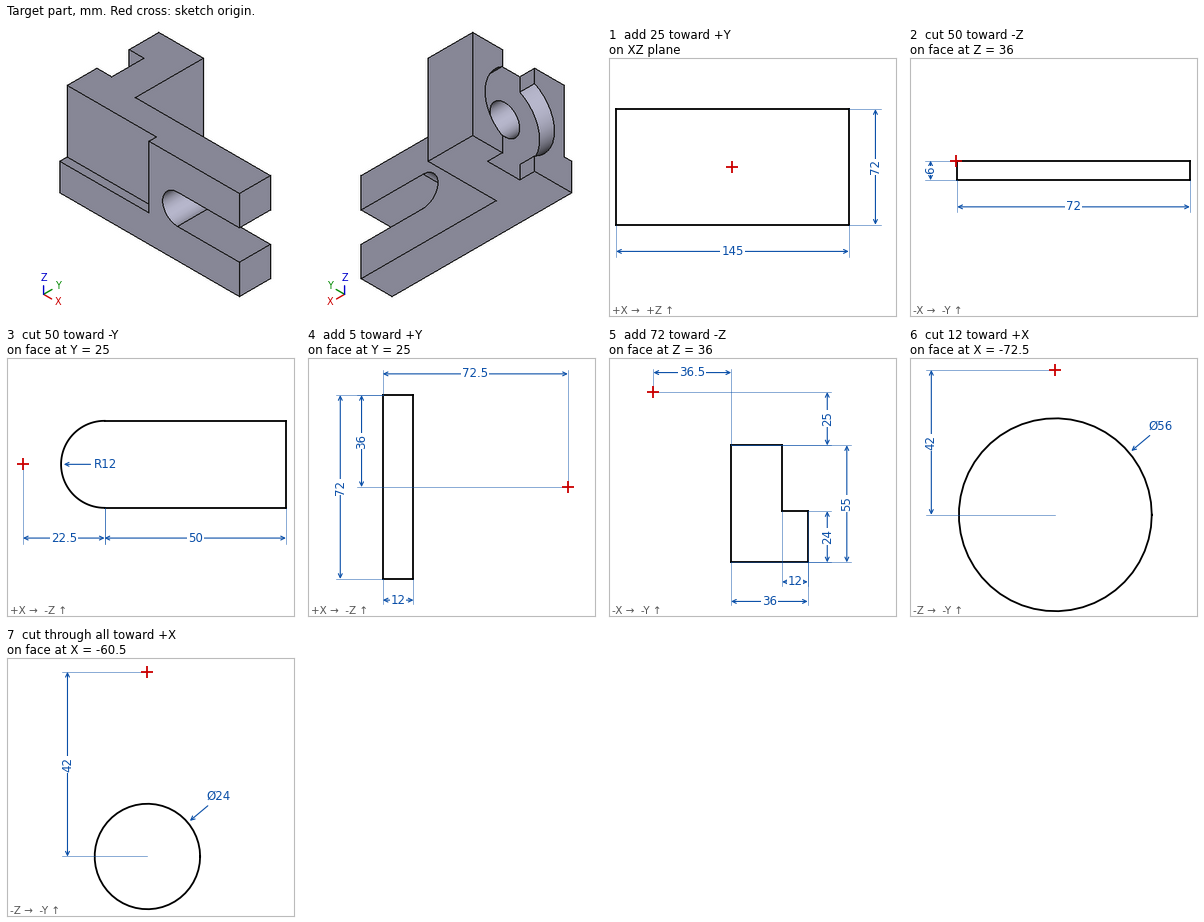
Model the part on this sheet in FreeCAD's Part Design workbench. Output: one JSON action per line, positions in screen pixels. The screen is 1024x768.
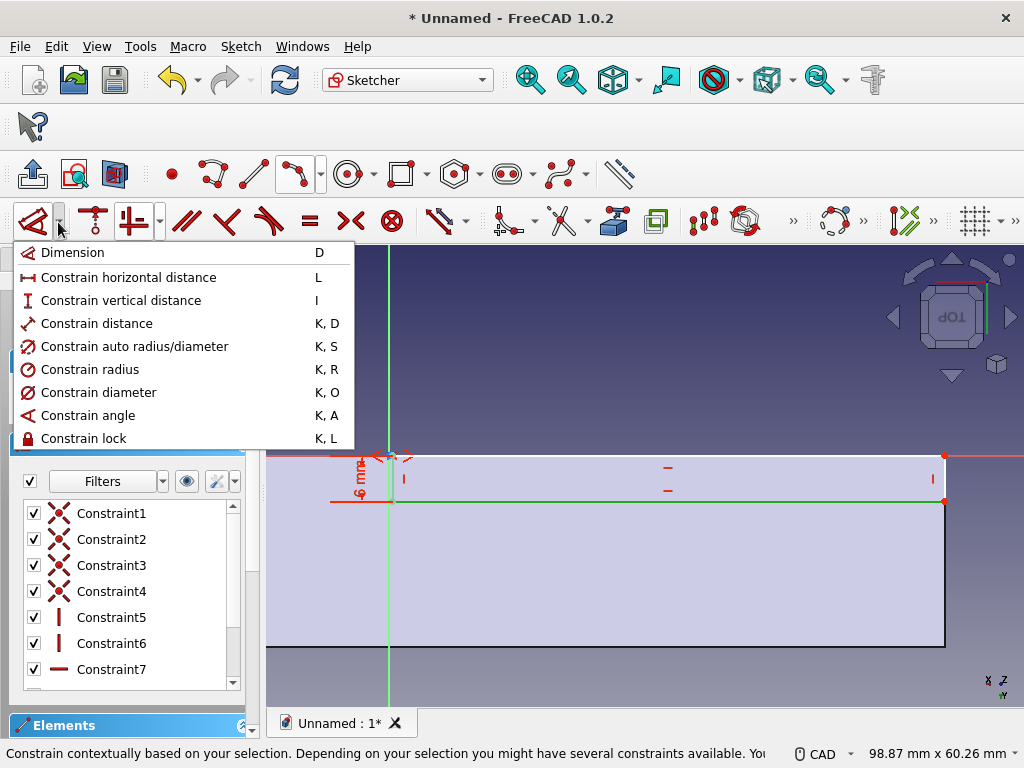
{"action": "left_click", "coordinate": [184, 278]}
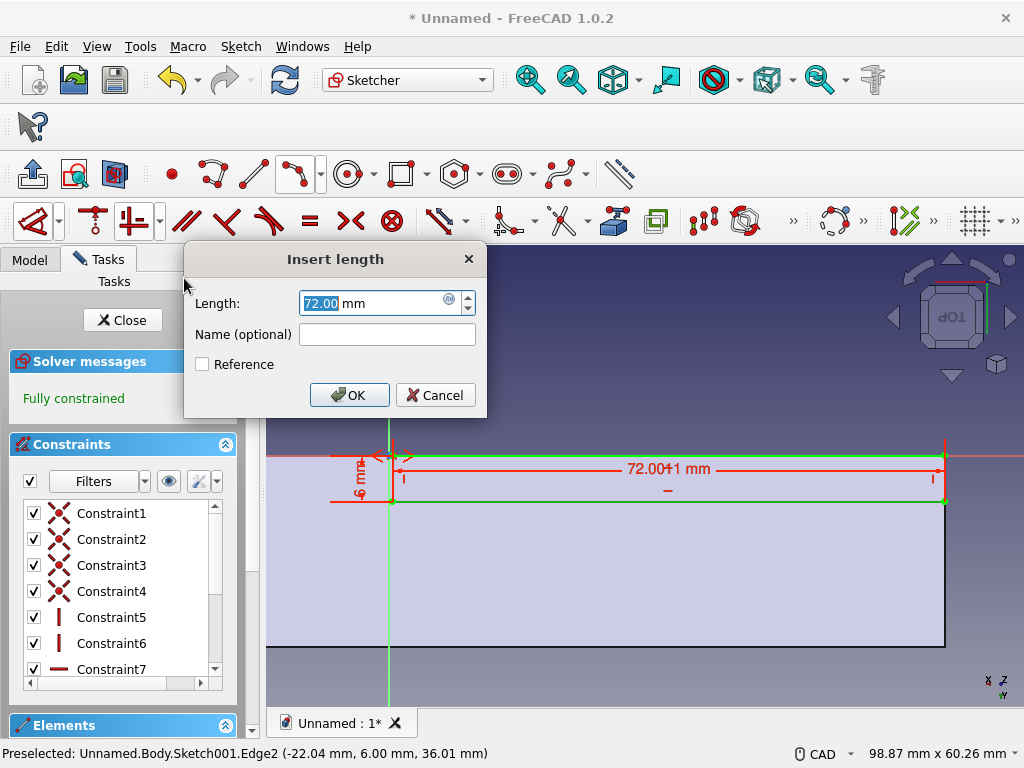
{"action": "type", "text": "72"}
{"action": "key", "text": "Return"}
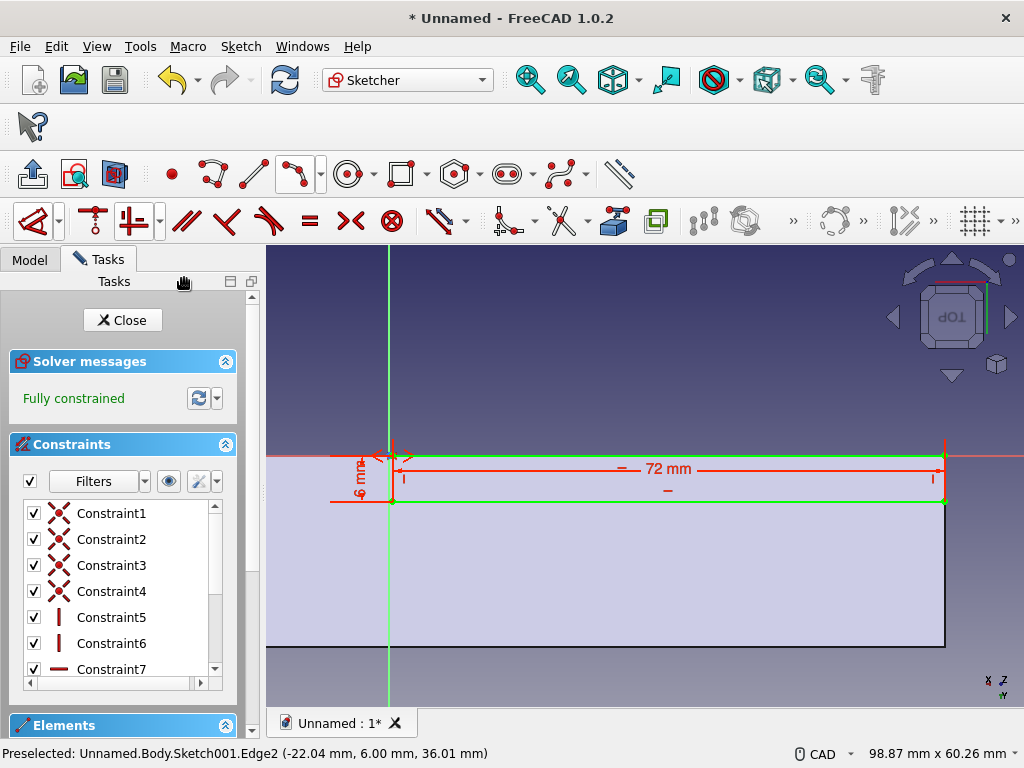
{"action": "left_click", "coordinate": [123, 320]}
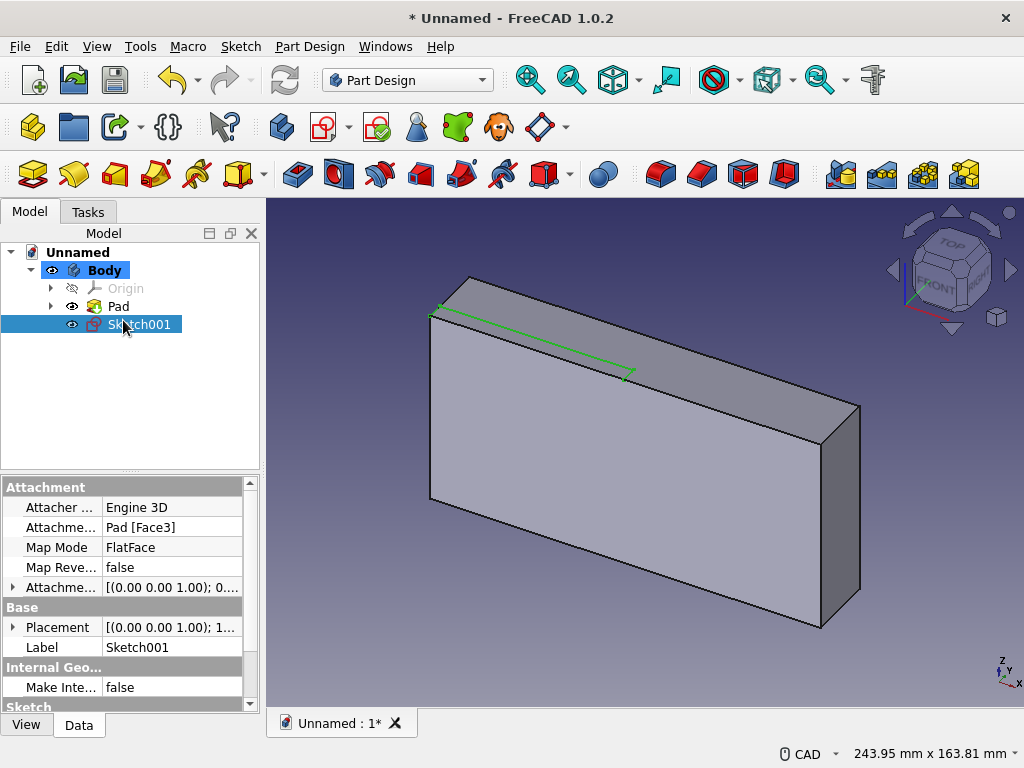
{"action": "left_click", "coordinate": [298, 174]}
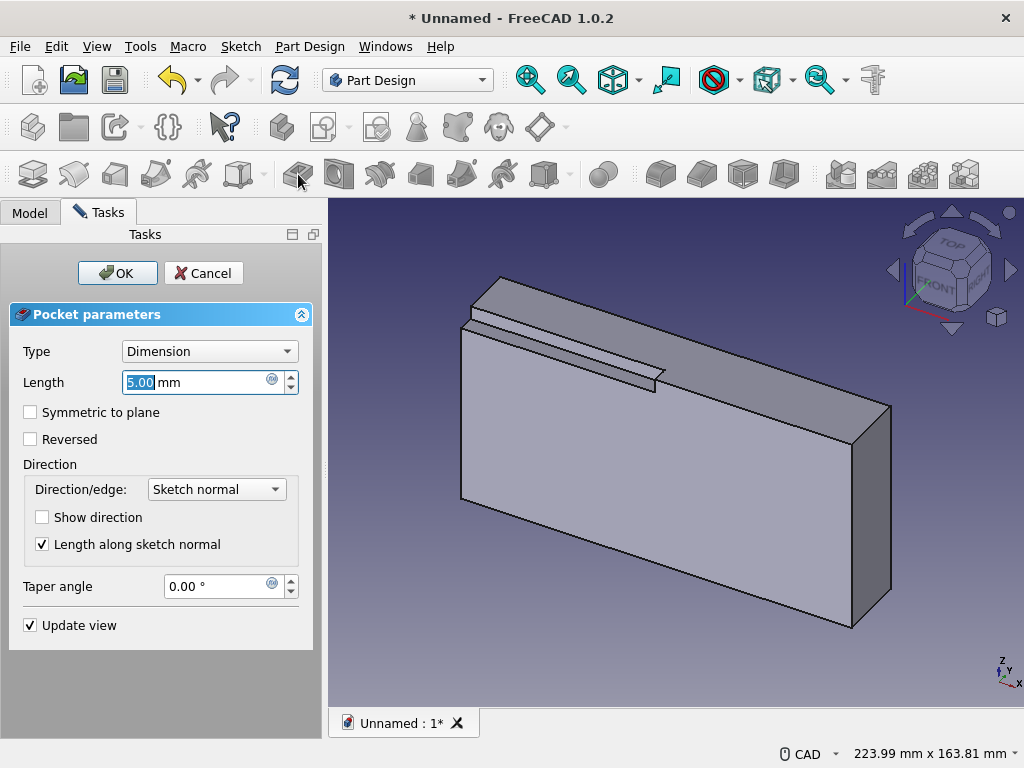
{"action": "type", "text": "50"}
{"action": "key", "text": "Tab"}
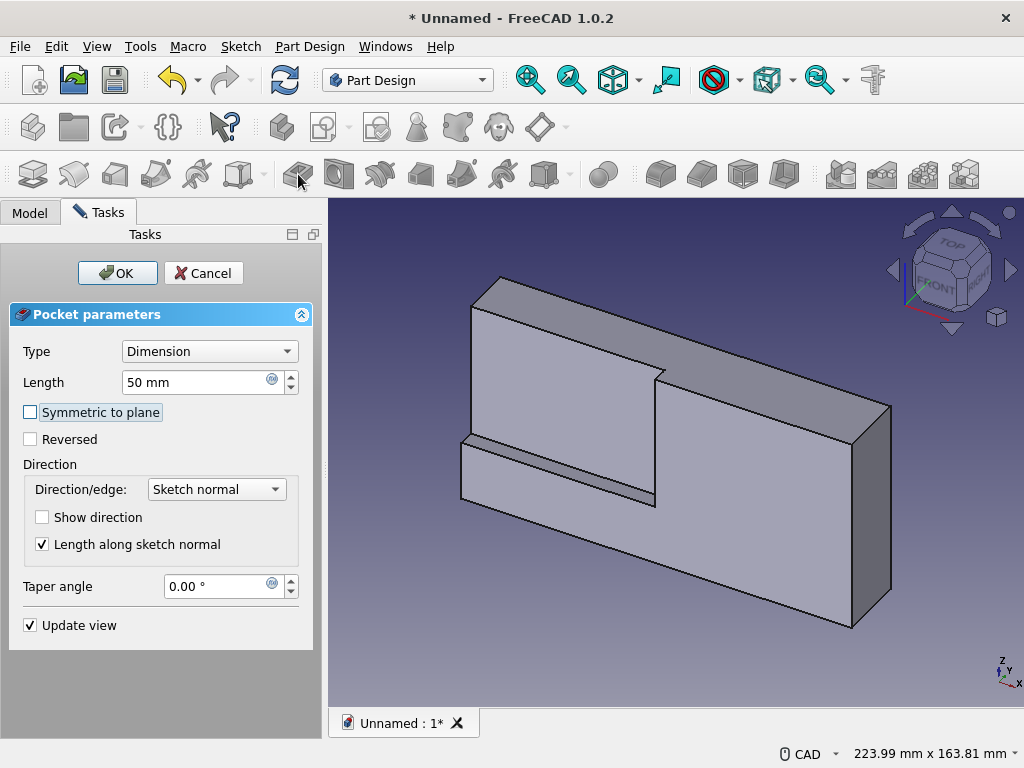
{"action": "left_click", "coordinate": [118, 273]}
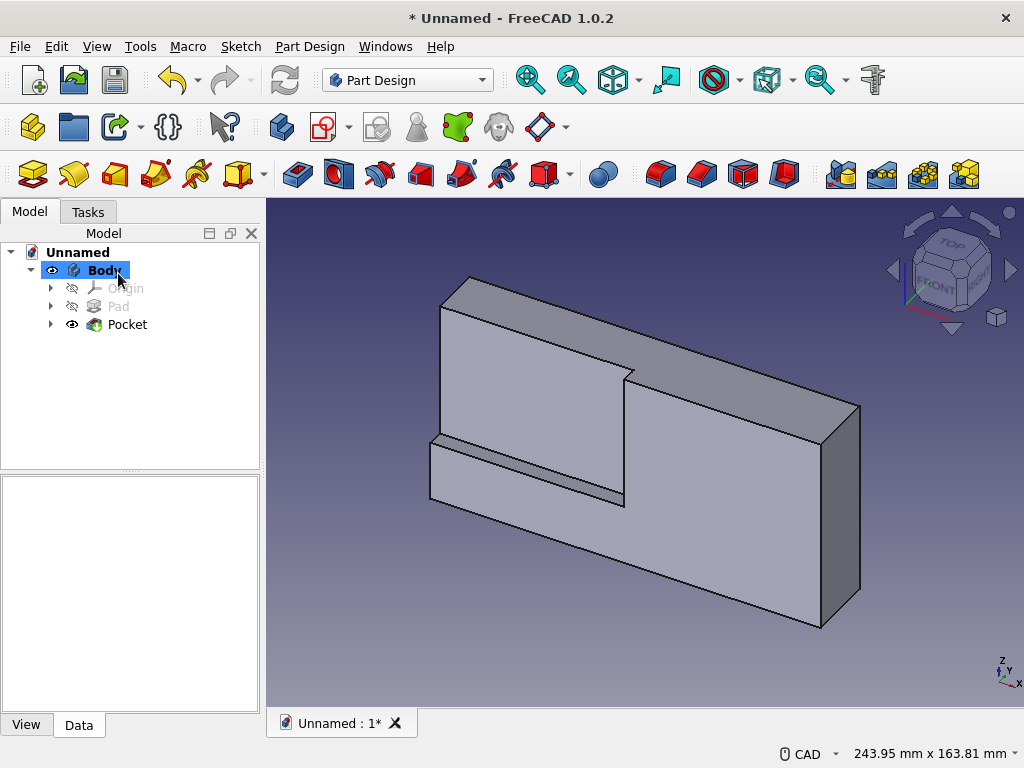
{"action": "key", "text": "4"}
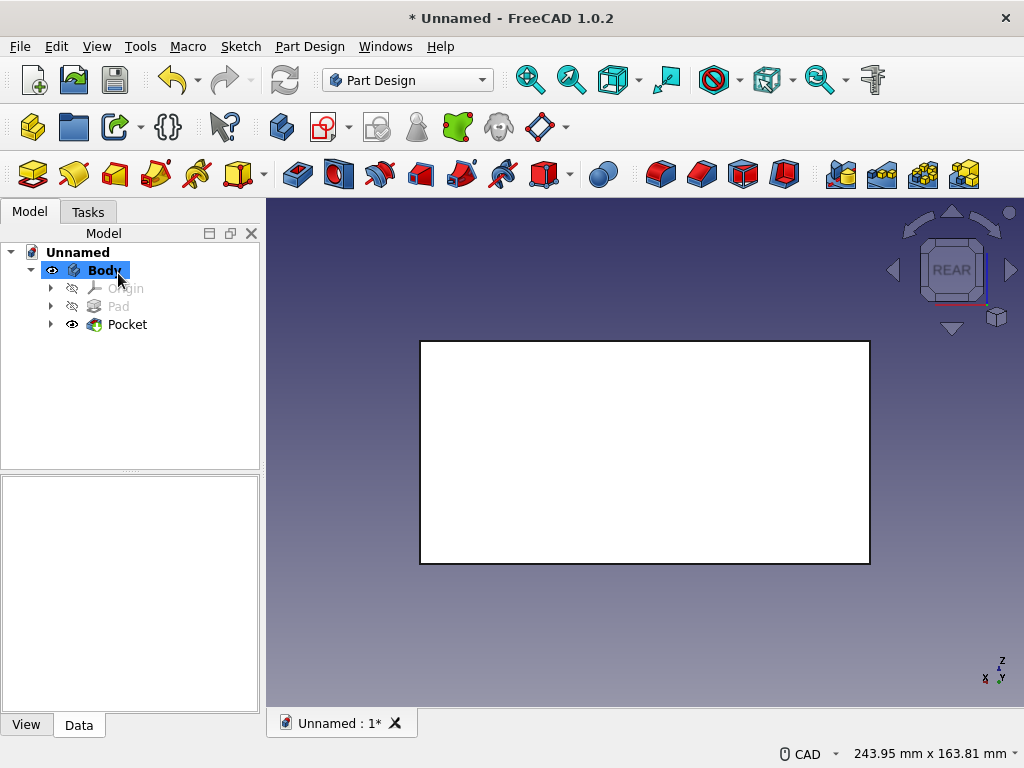
{"action": "left_click", "coordinate": [581, 452]}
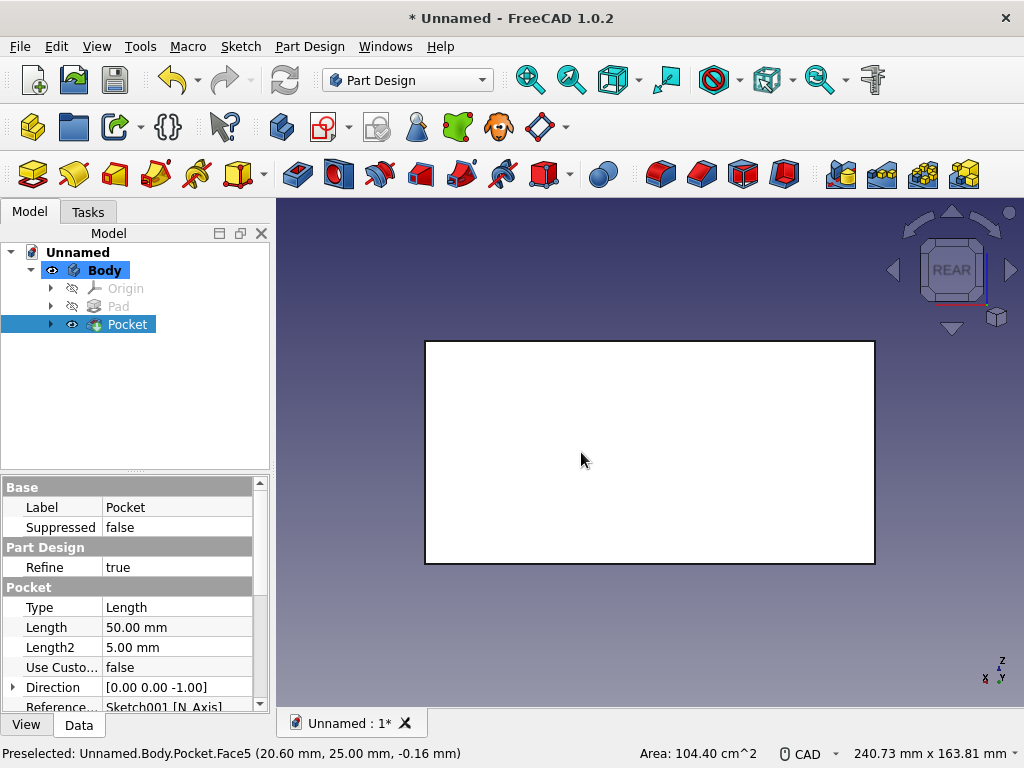
{"action": "left_click", "coordinate": [322, 128]}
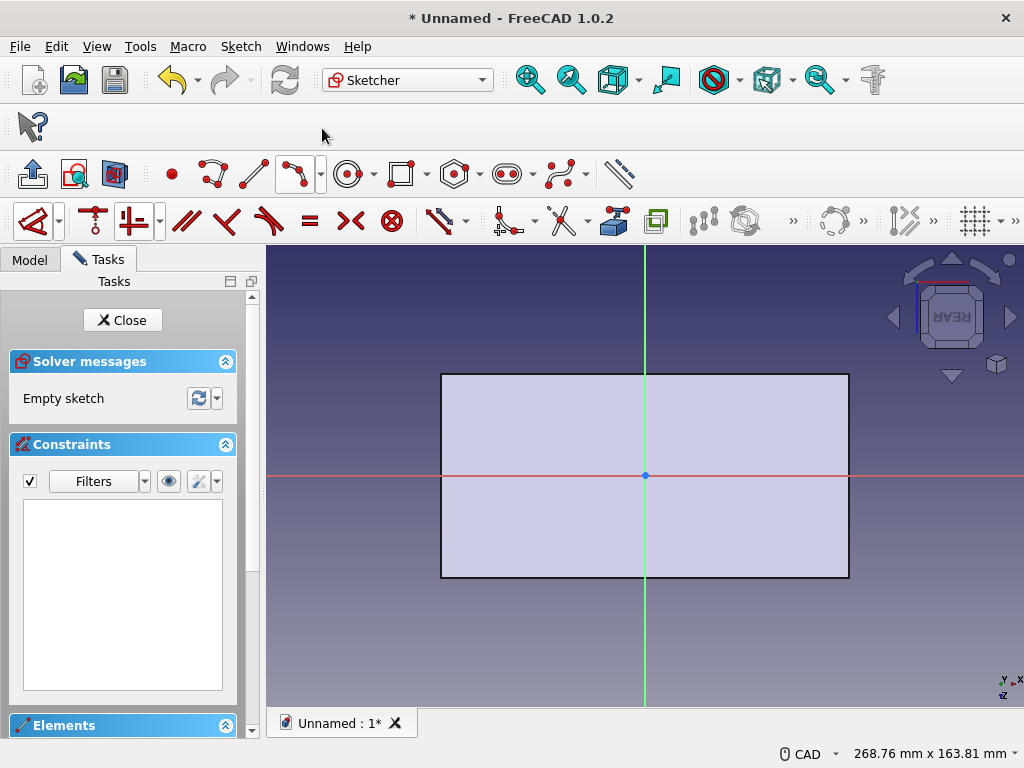
{"action": "scroll", "coordinate": [576, 476], "scroll_direction": "down", "scroll_amount": 5}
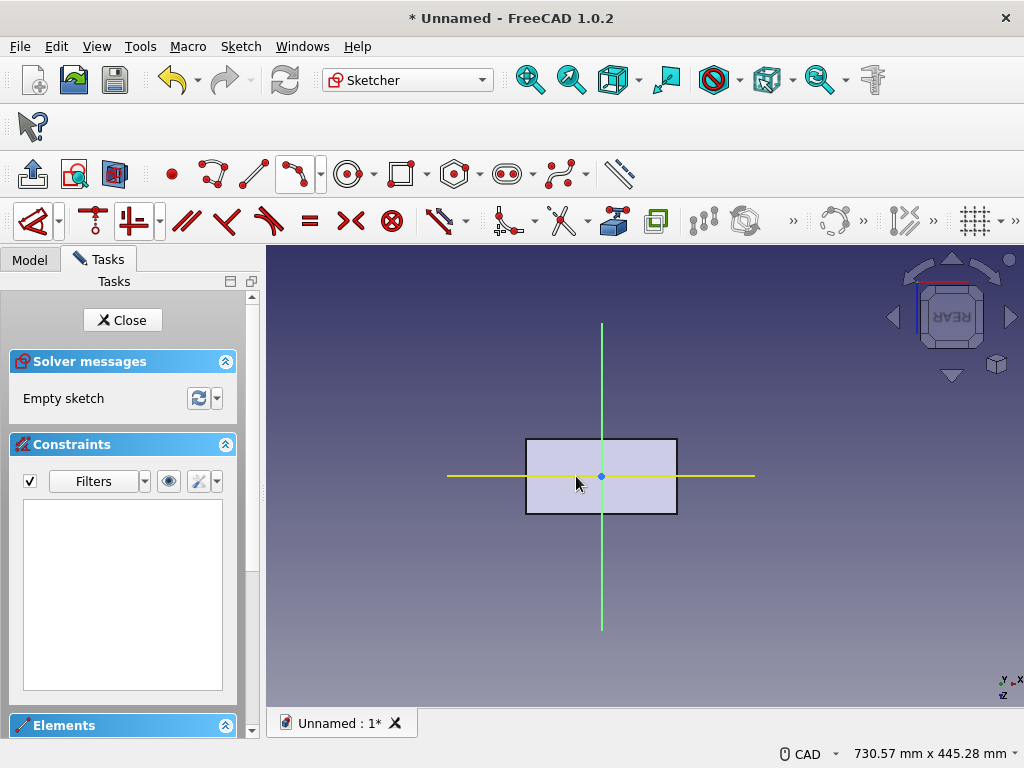
{"action": "scroll", "coordinate": [655, 476], "scroll_direction": "up", "scroll_amount": 8}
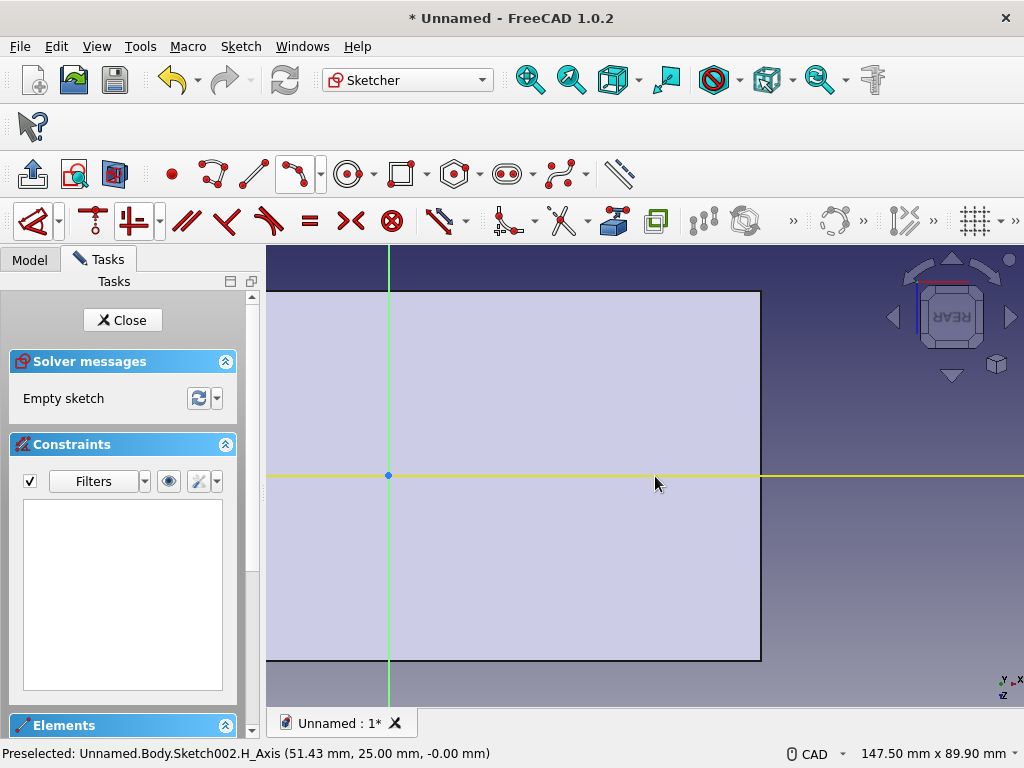
{"action": "left_click", "coordinate": [213, 174]}